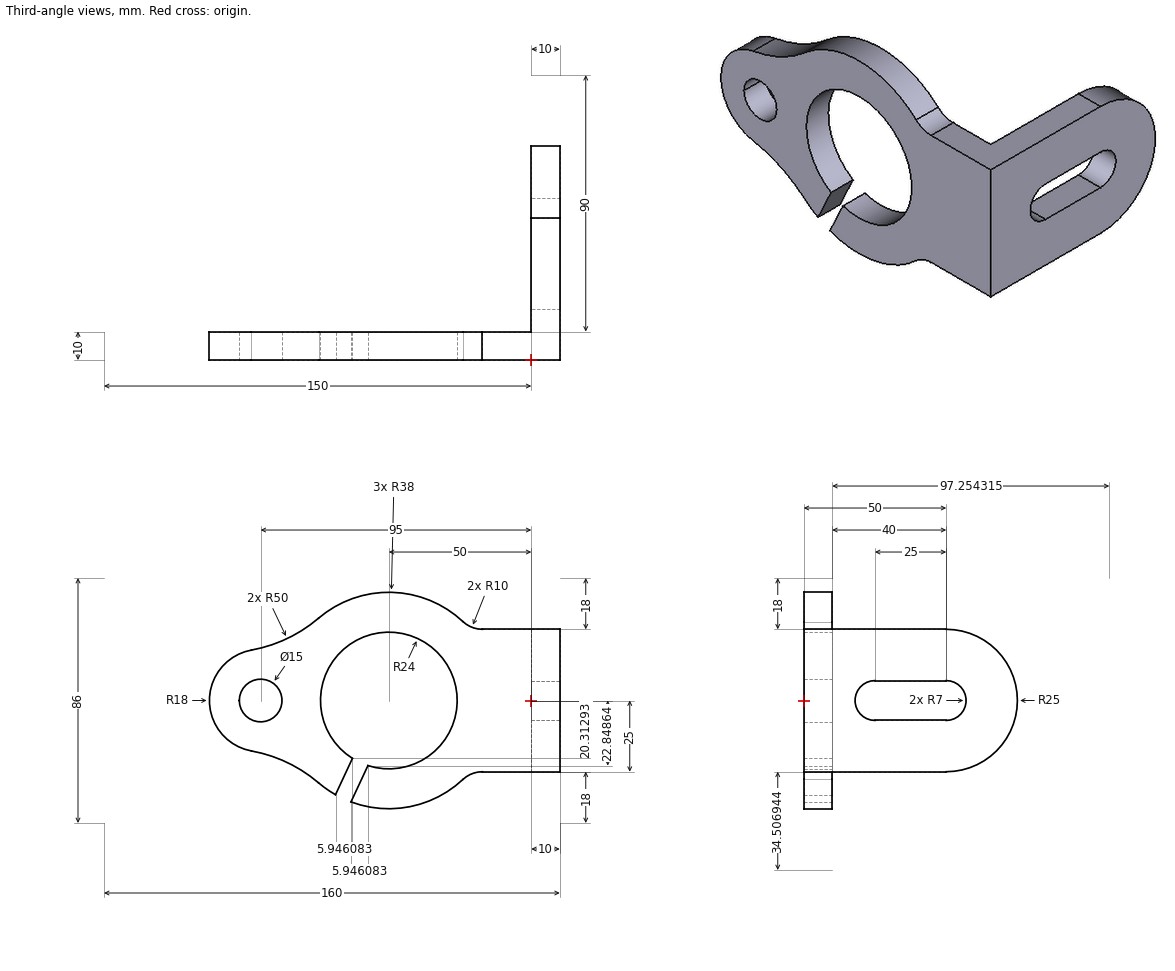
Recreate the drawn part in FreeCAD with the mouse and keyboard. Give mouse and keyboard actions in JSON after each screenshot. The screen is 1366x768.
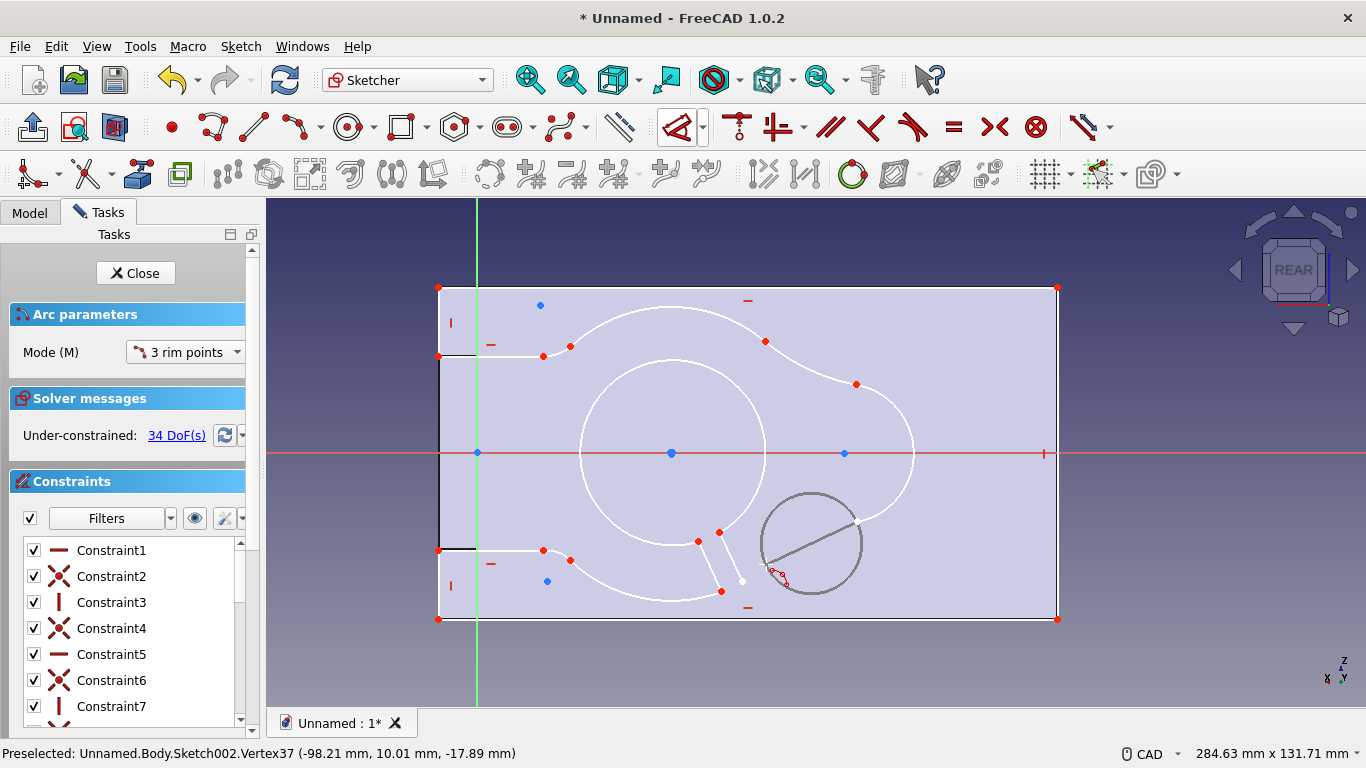
{"action": "scroll", "coordinate": [809, 537], "scroll_direction": "up", "scroll_amount": 5}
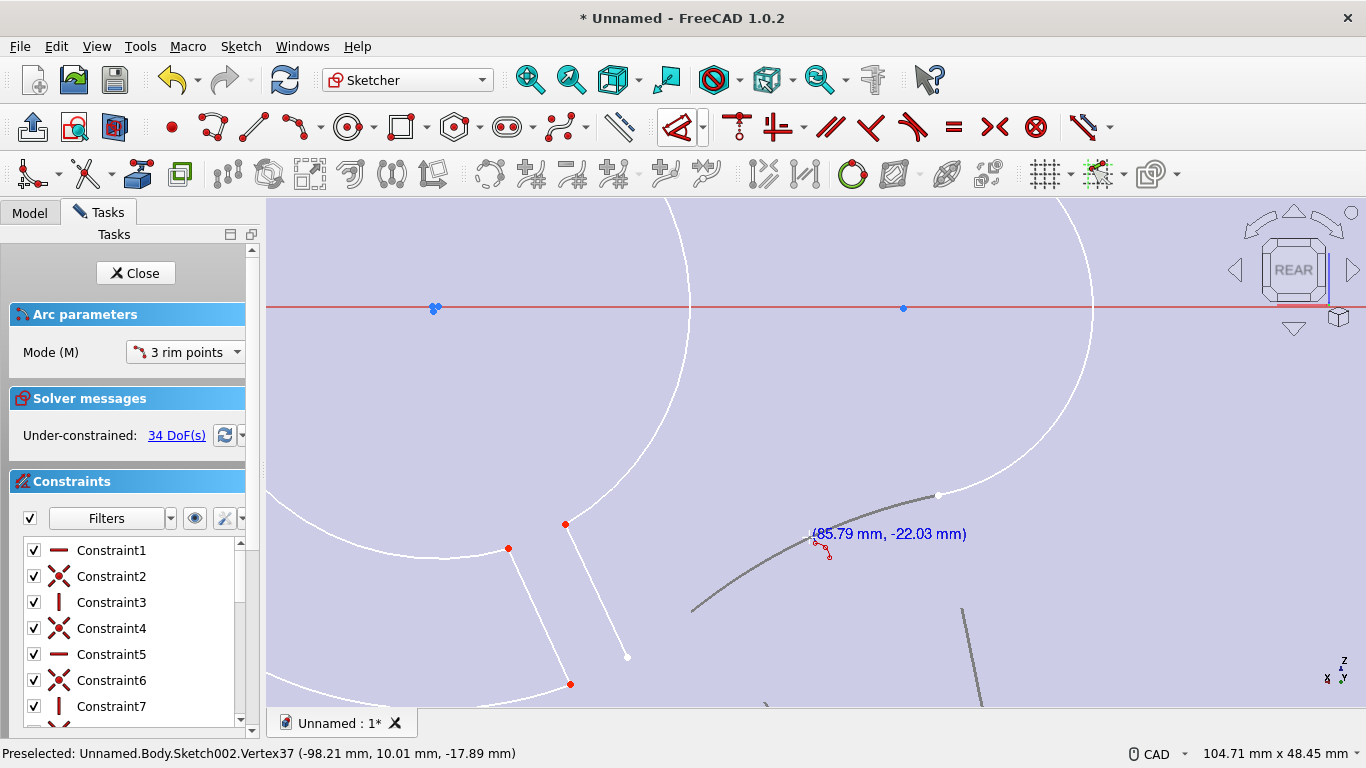
{"action": "left_click", "coordinate": [807, 535]}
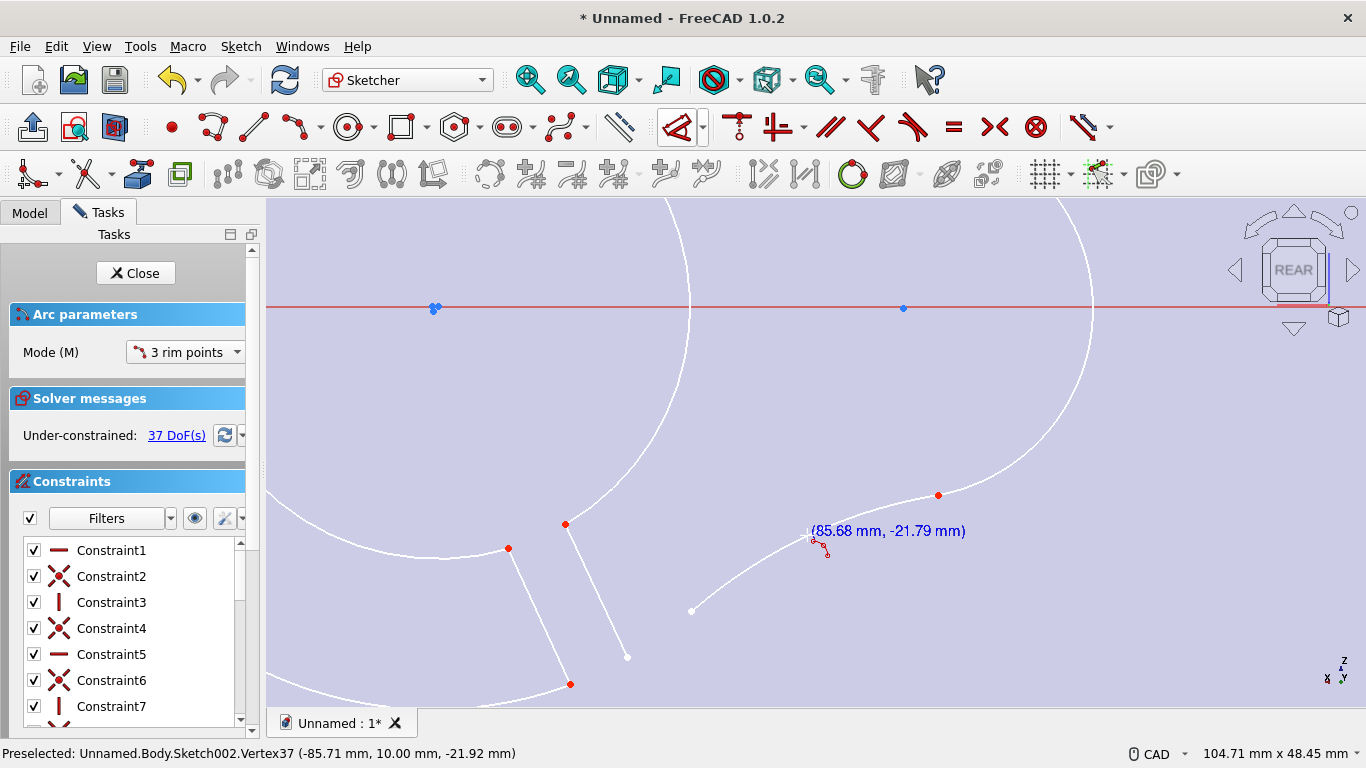
{"action": "left_click", "coordinate": [691, 612]}
{"action": "left_click", "coordinate": [628, 658]}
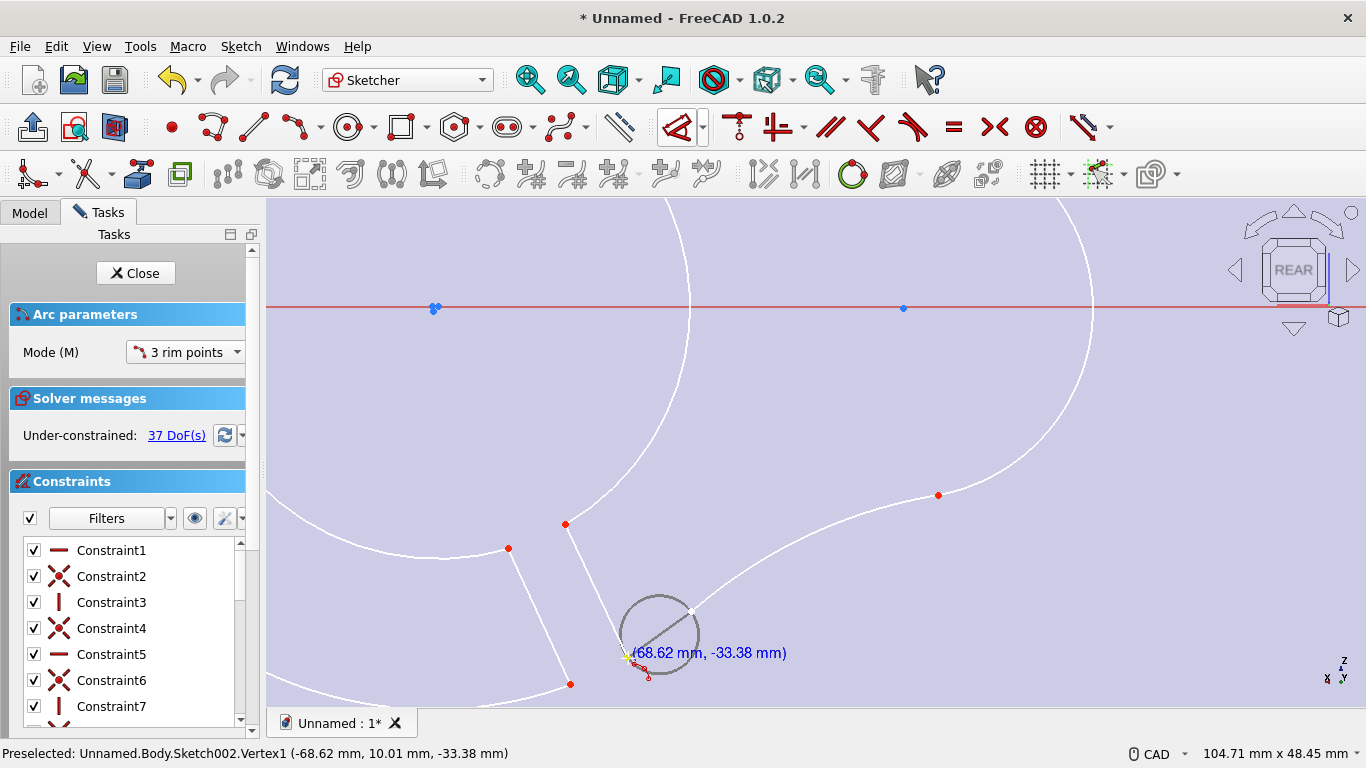
{"action": "scroll", "coordinate": [661, 634], "scroll_direction": "up", "scroll_amount": 11}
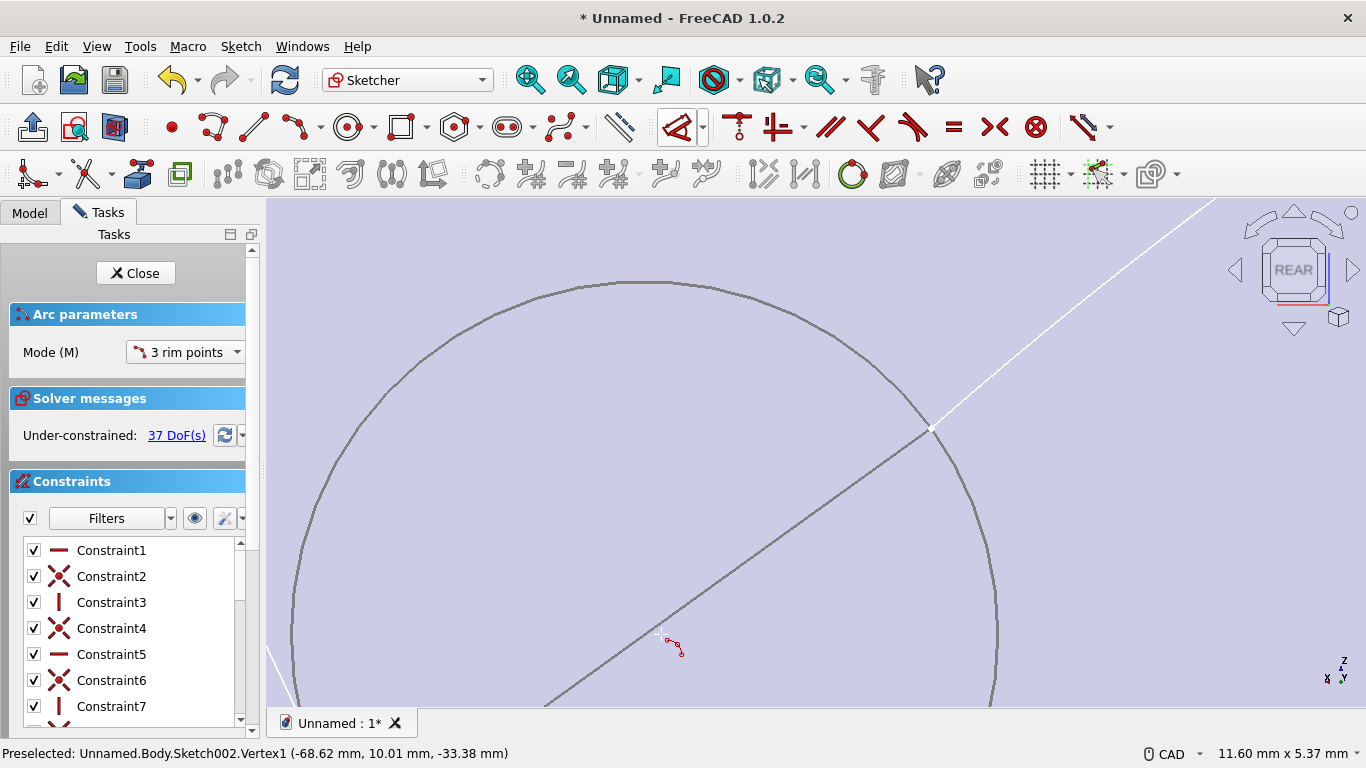
{"action": "left_click", "coordinate": [660, 627]}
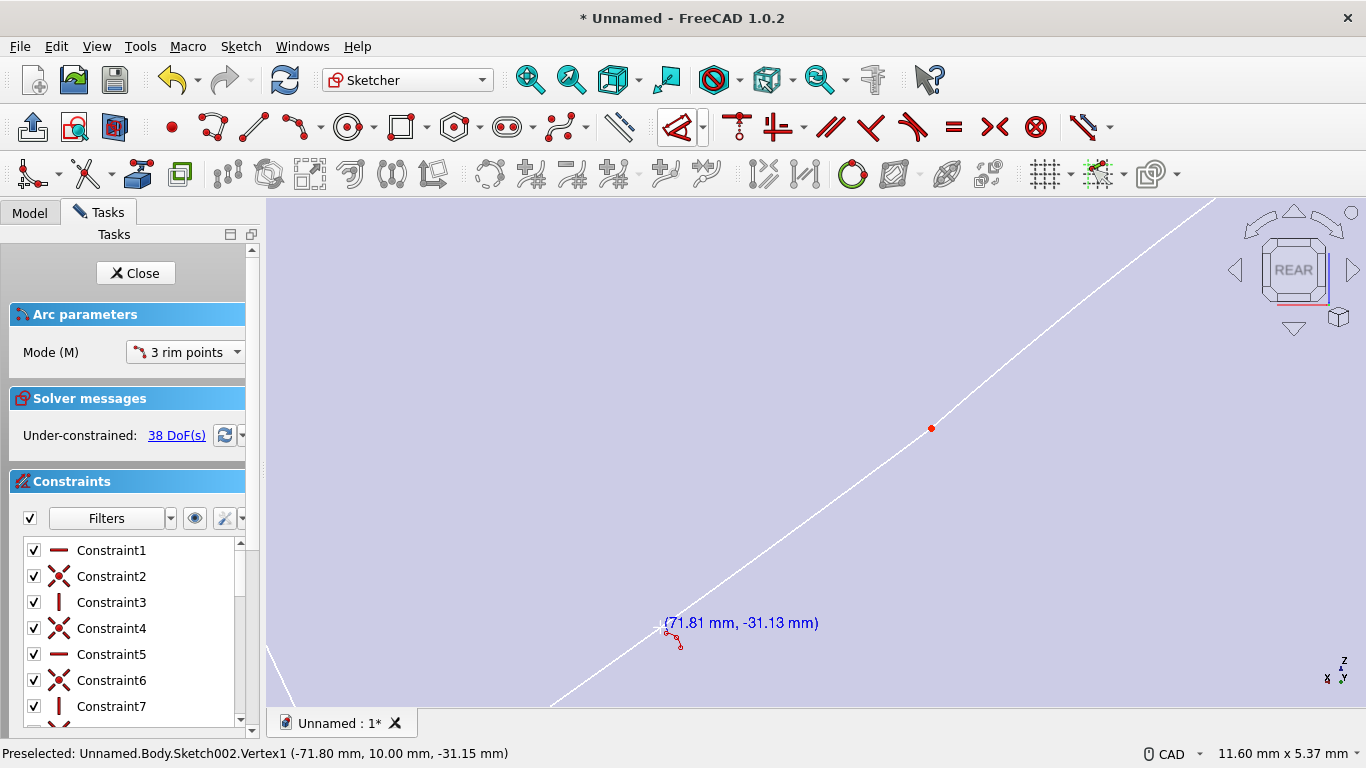
{"action": "left_click", "coordinate": [348, 128]}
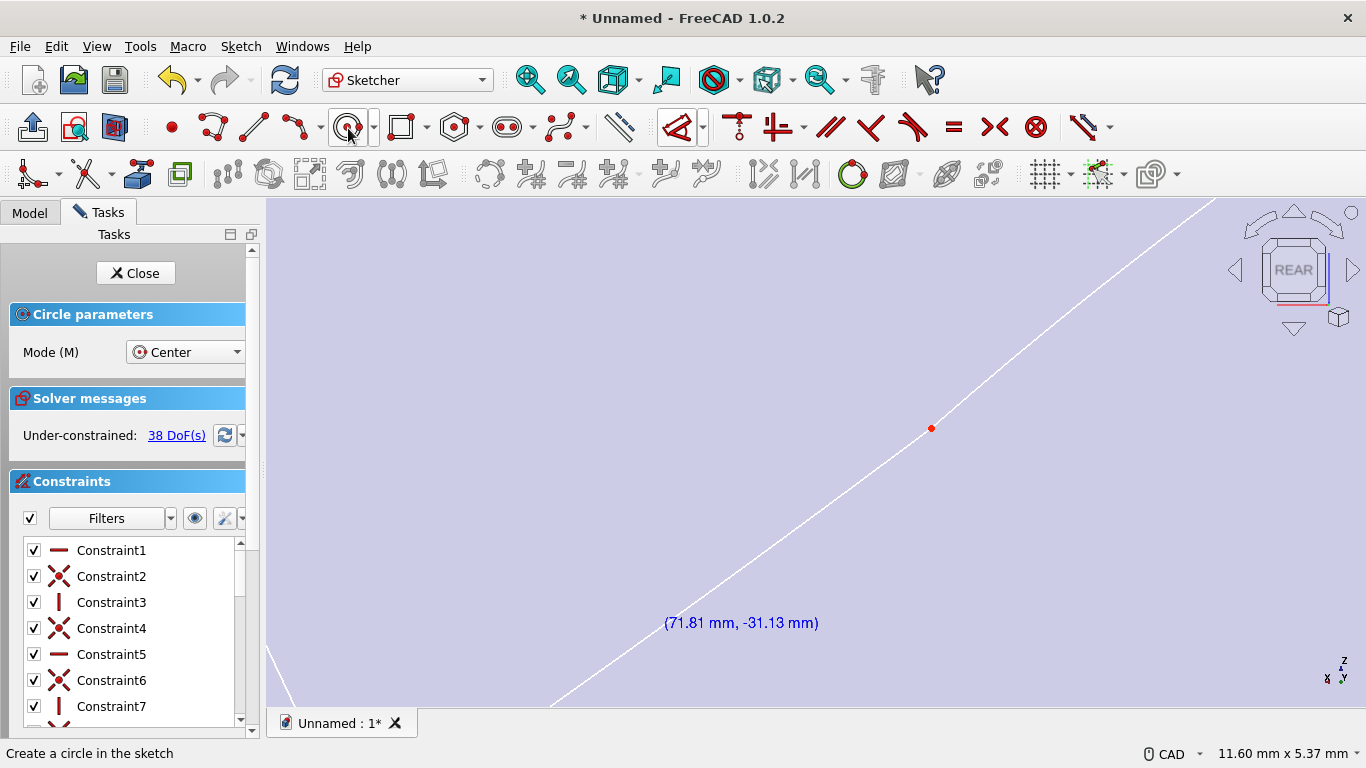
{"action": "scroll", "coordinate": [758, 570], "scroll_direction": "down", "scroll_amount": 16}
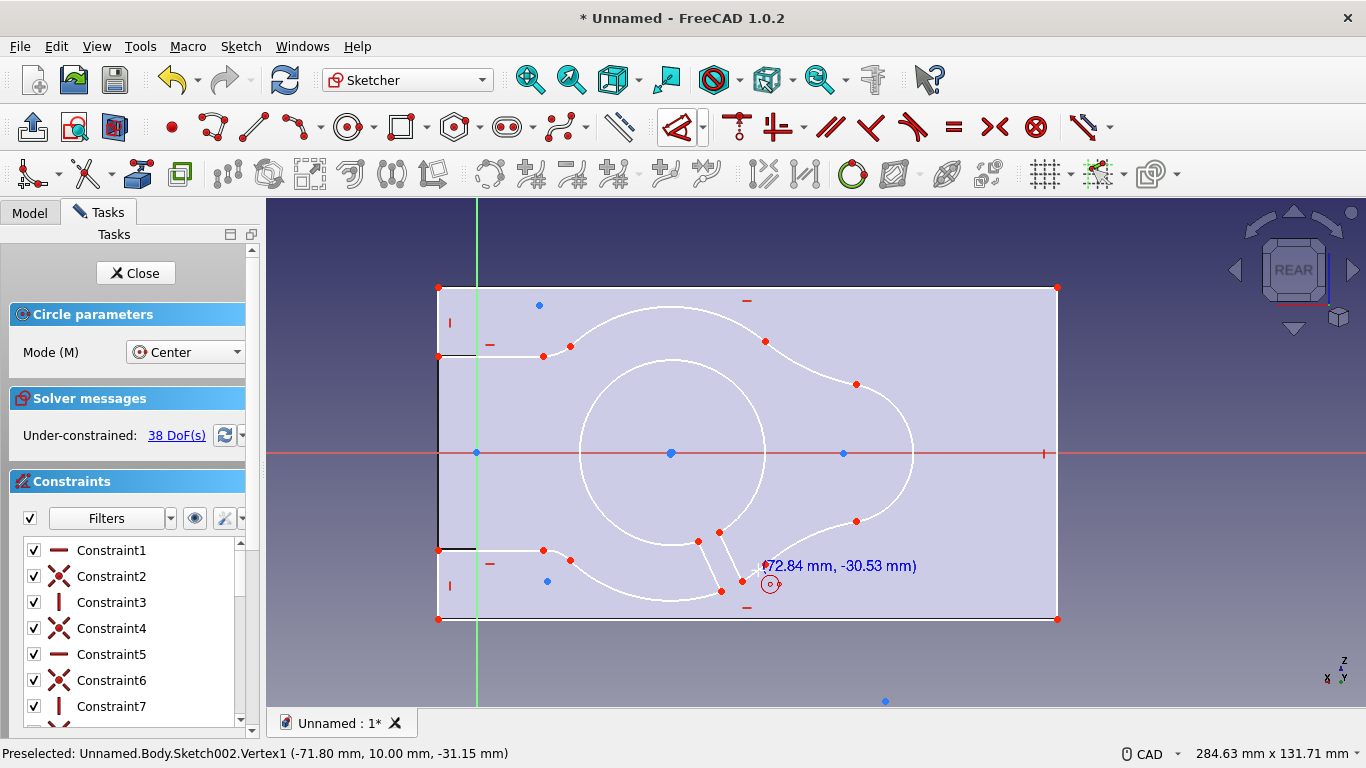
{"action": "left_click", "coordinate": [844, 453]}
{"action": "left_click", "coordinate": [865, 432]}
{"action": "key", "text": "Escape"}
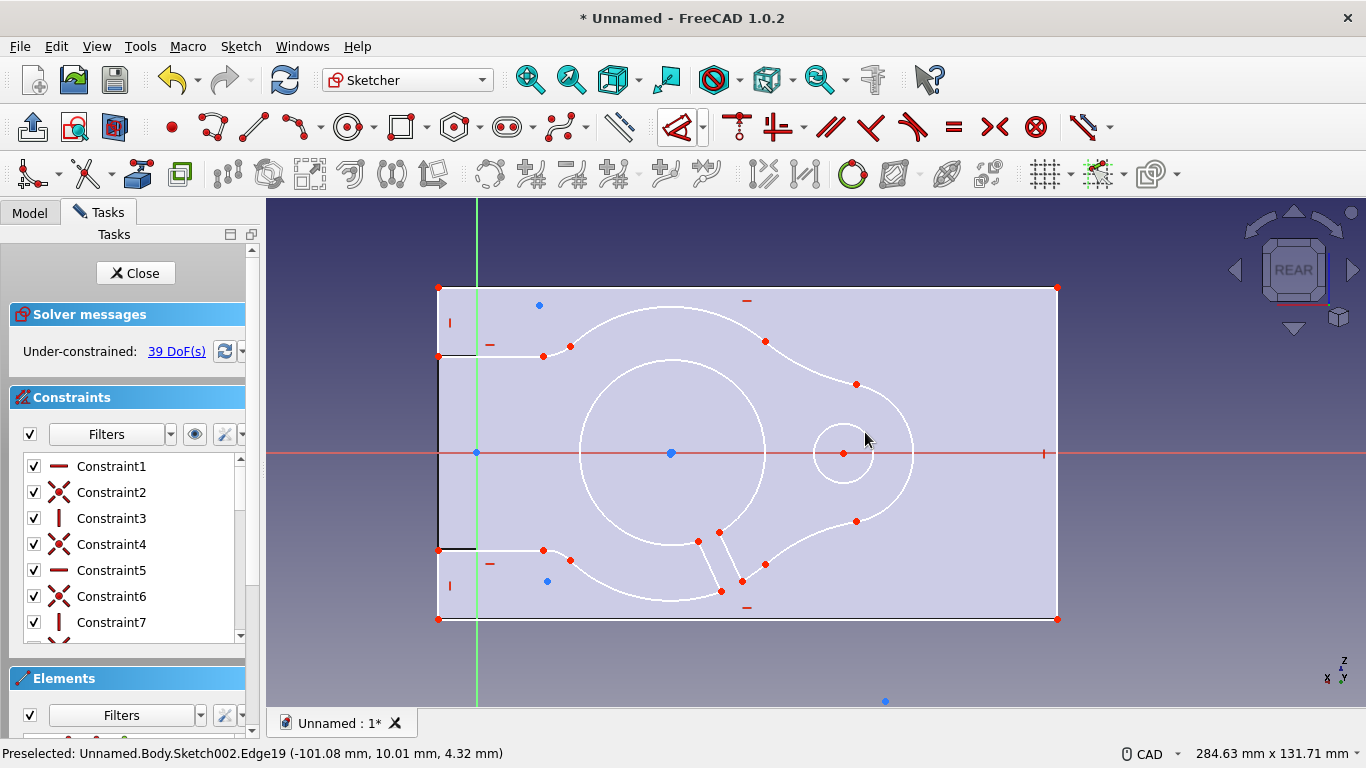
{"action": "left_click", "coordinate": [512, 551]}